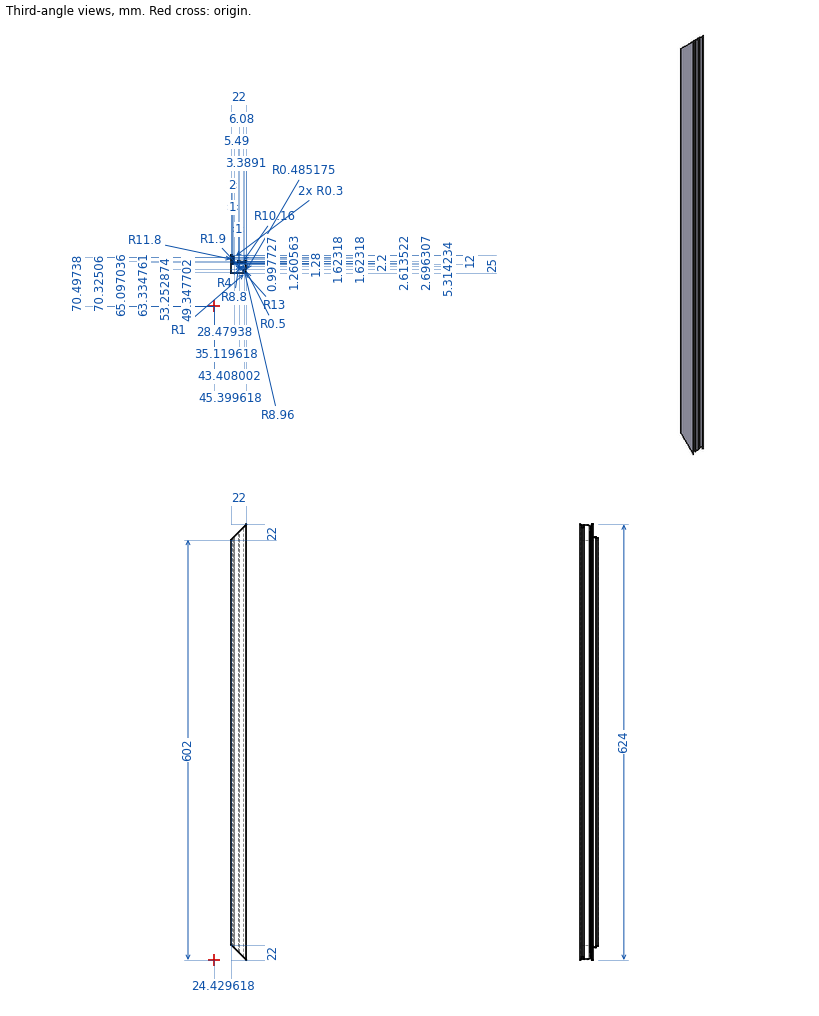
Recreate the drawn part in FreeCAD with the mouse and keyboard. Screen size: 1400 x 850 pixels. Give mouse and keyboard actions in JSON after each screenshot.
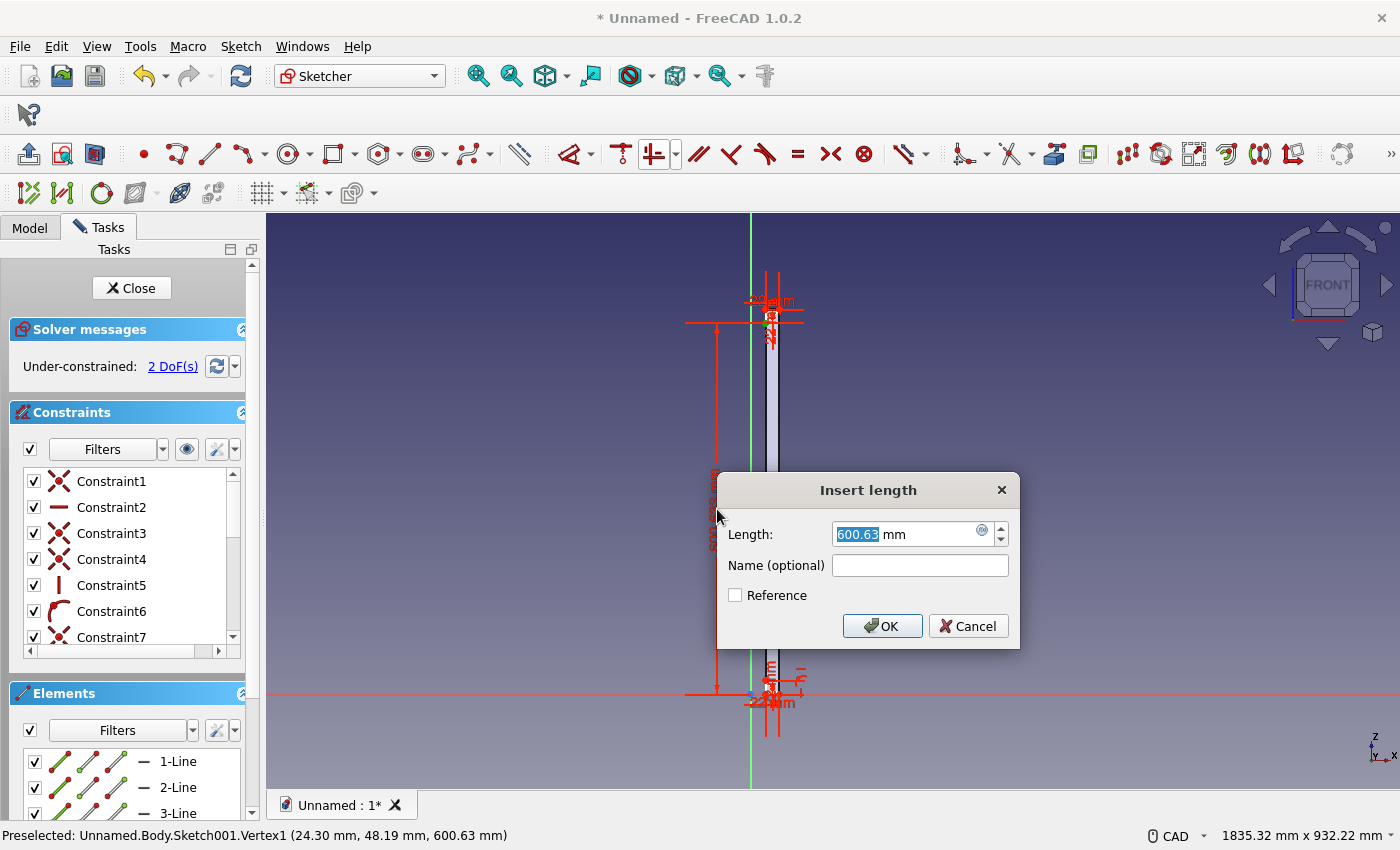
{"action": "type", "text": "602"}
{"action": "key", "text": "Return"}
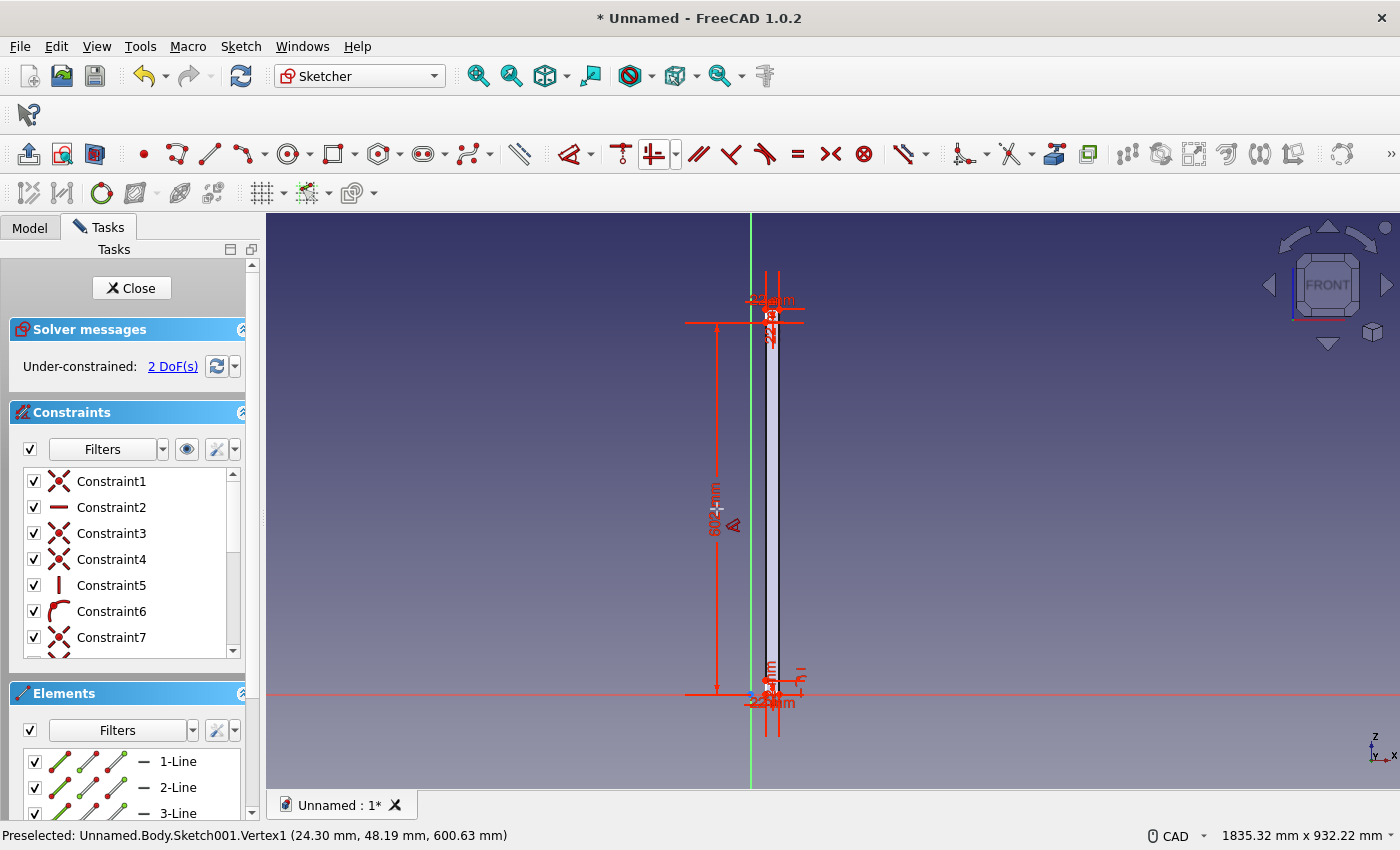
{"action": "scroll", "coordinate": [766, 323], "scroll_direction": "up", "scroll_amount": 5}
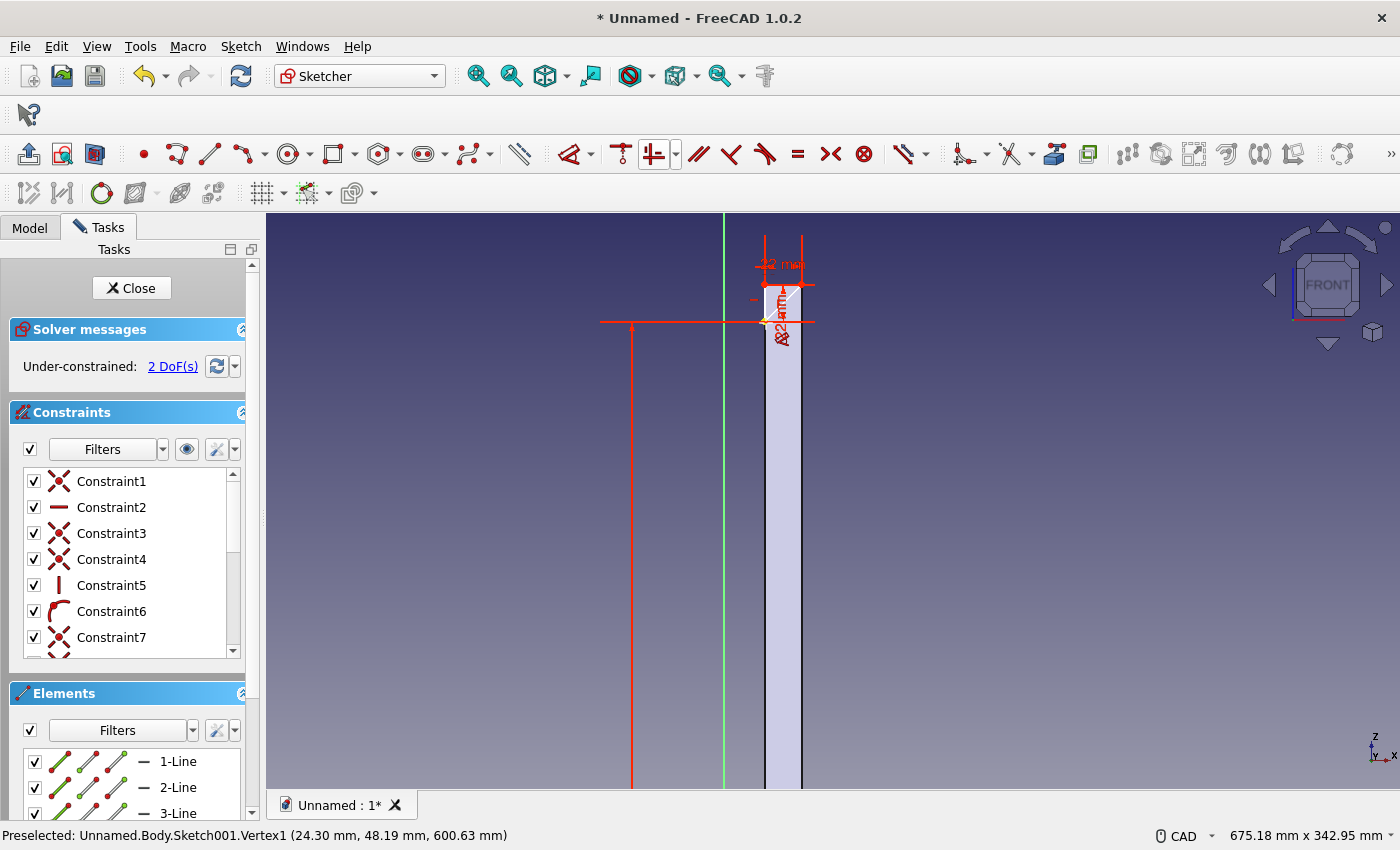
{"action": "left_click", "coordinate": [765, 322]}
{"action": "left_click", "coordinate": [744, 288]}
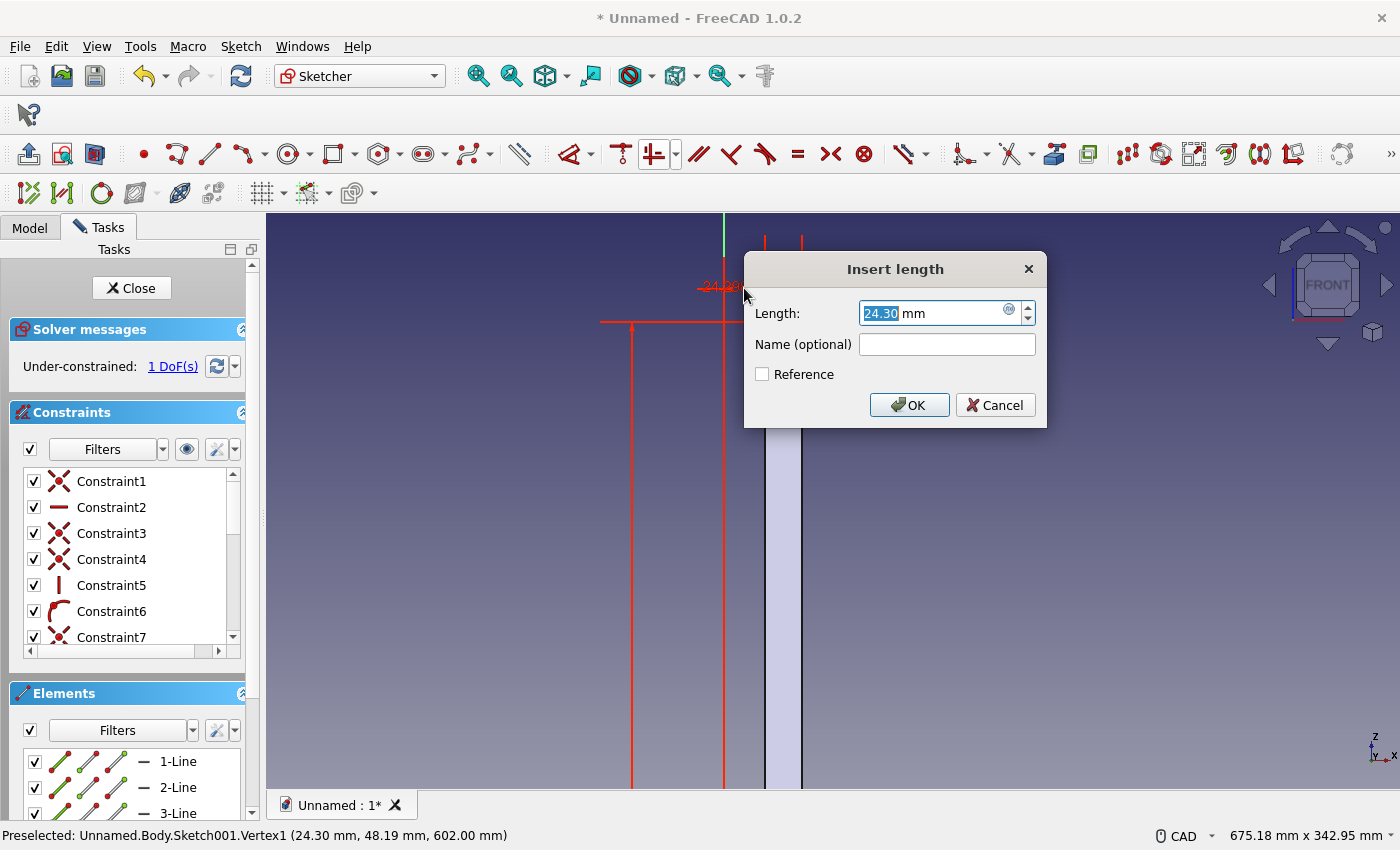
{"action": "type", "text": "24.429618"}
{"action": "key", "text": "Return"}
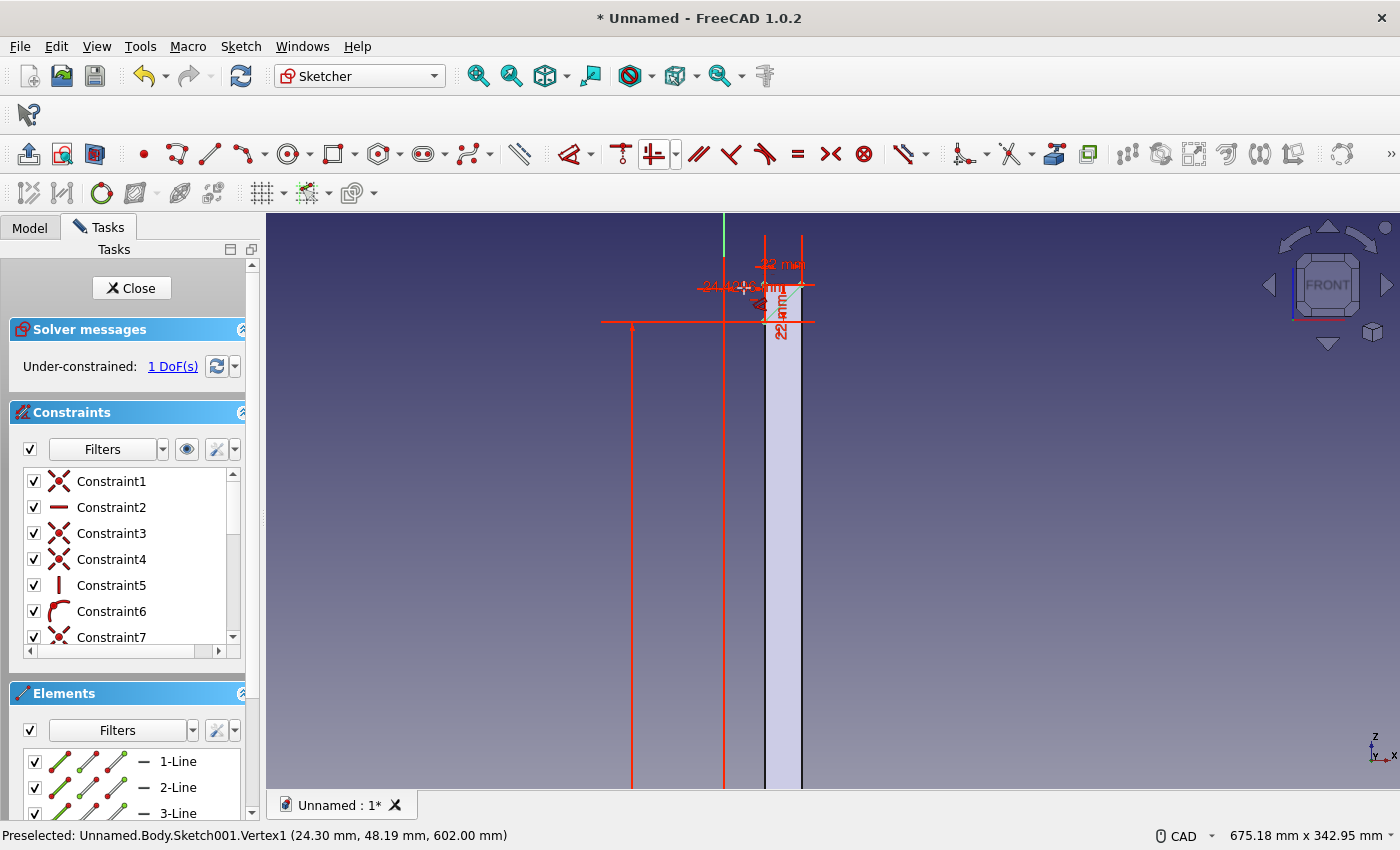
{"action": "scroll", "coordinate": [766, 322], "scroll_direction": "down", "scroll_amount": 5}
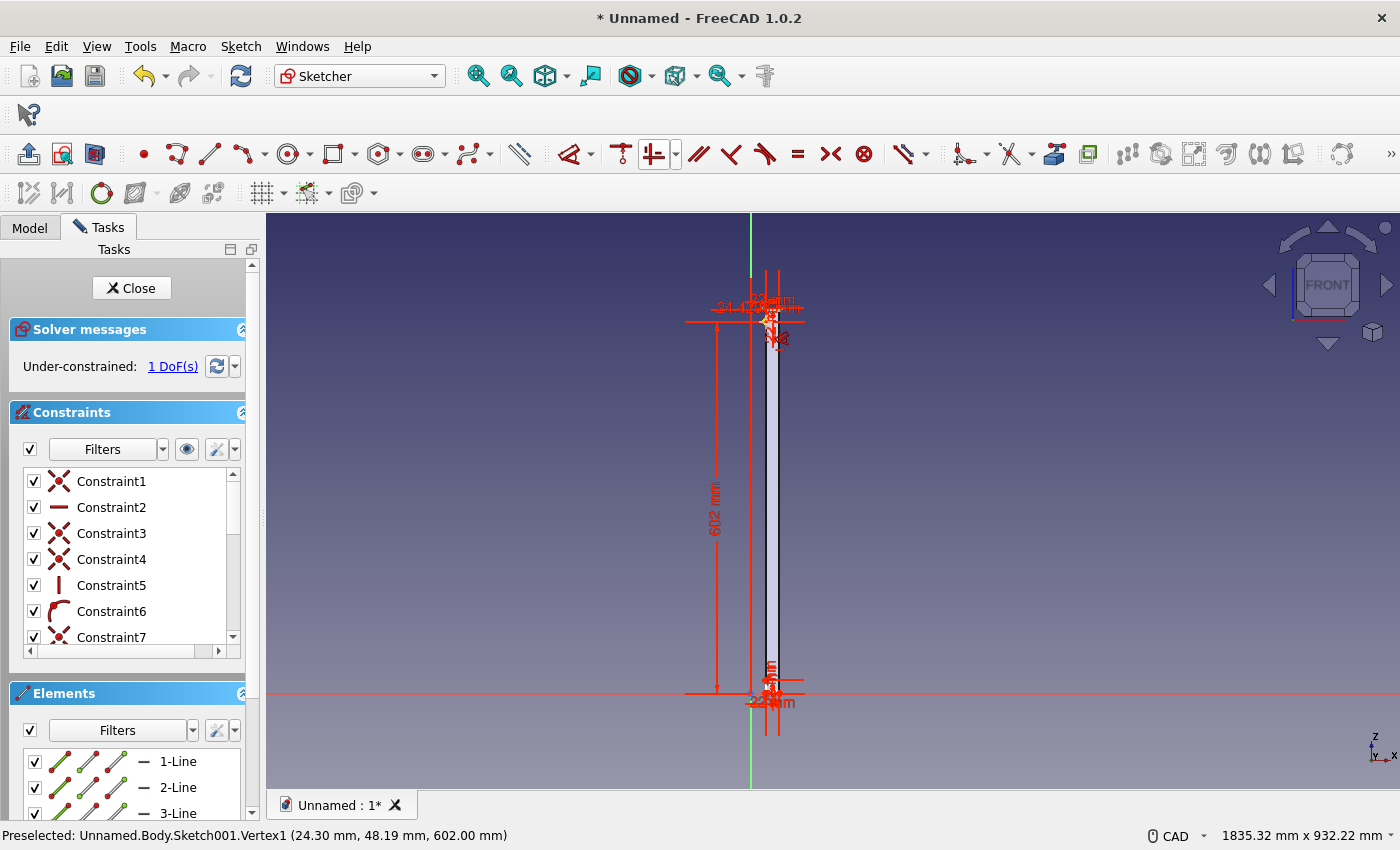
{"action": "scroll", "coordinate": [766, 694], "scroll_direction": "up", "scroll_amount": 5}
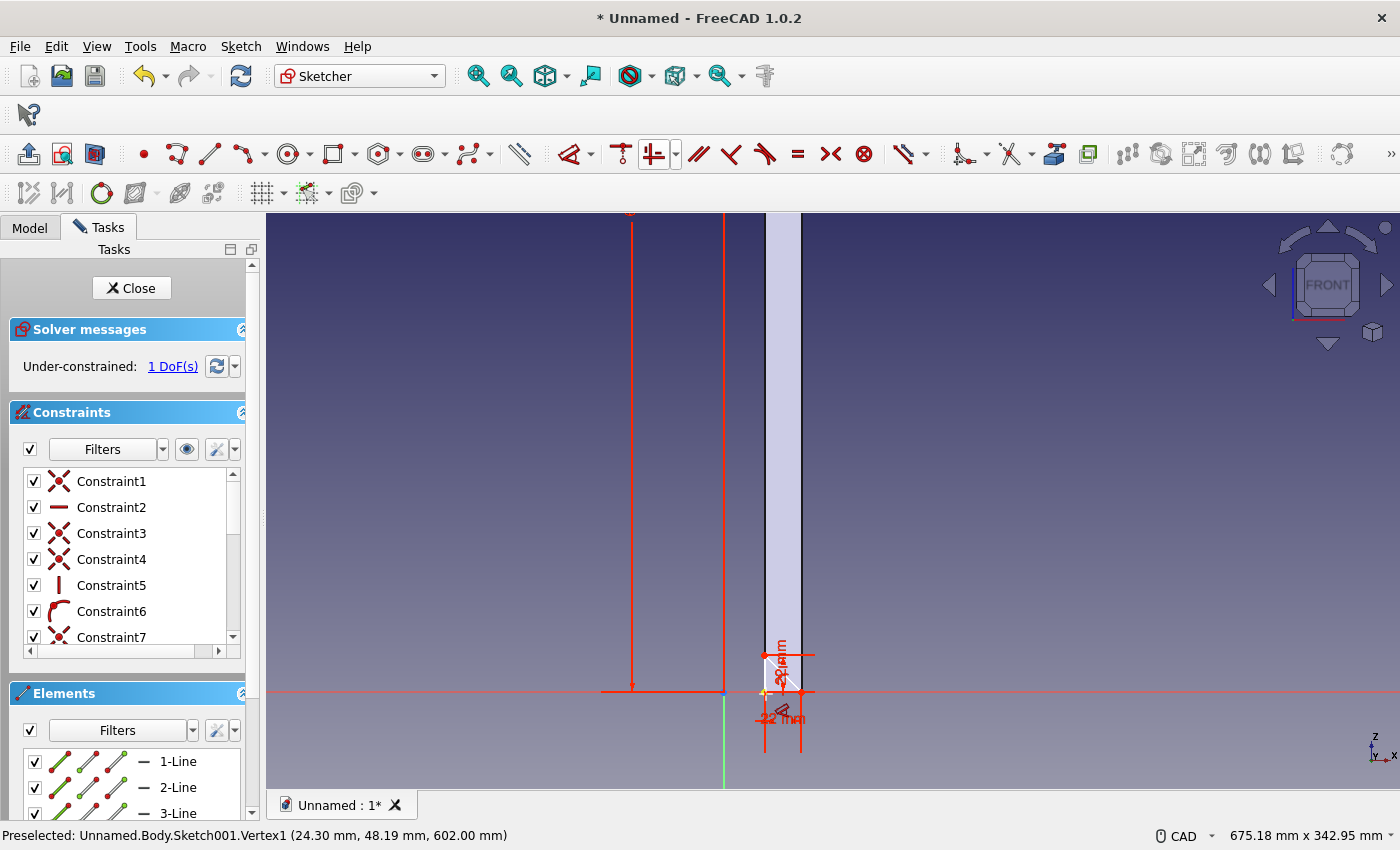
{"action": "left_click", "coordinate": [765, 692]}
{"action": "left_click", "coordinate": [744, 750]}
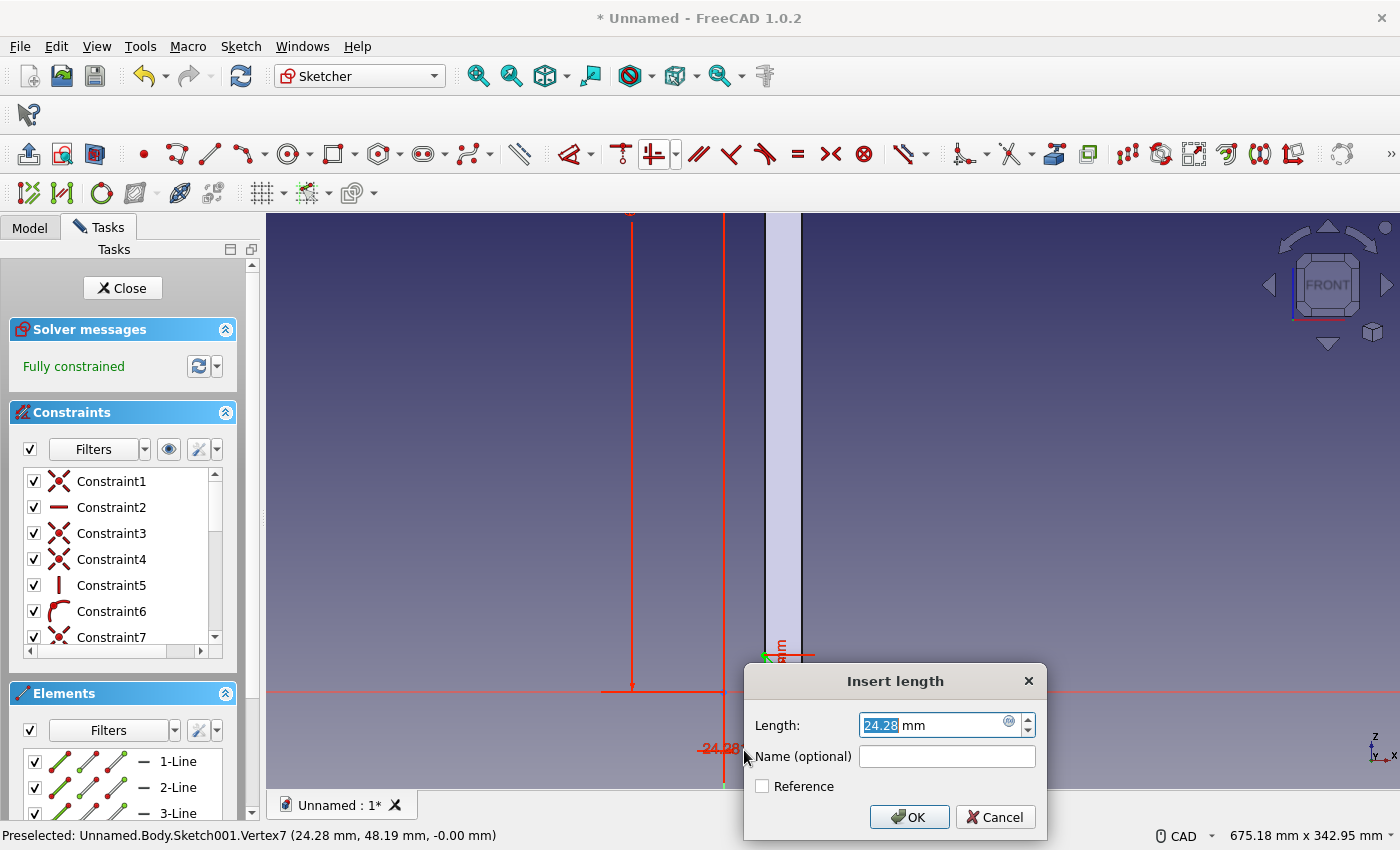
{"action": "type", "text": "24.429618"}
{"action": "key", "text": "Return"}
{"action": "key", "text": "Escape"}